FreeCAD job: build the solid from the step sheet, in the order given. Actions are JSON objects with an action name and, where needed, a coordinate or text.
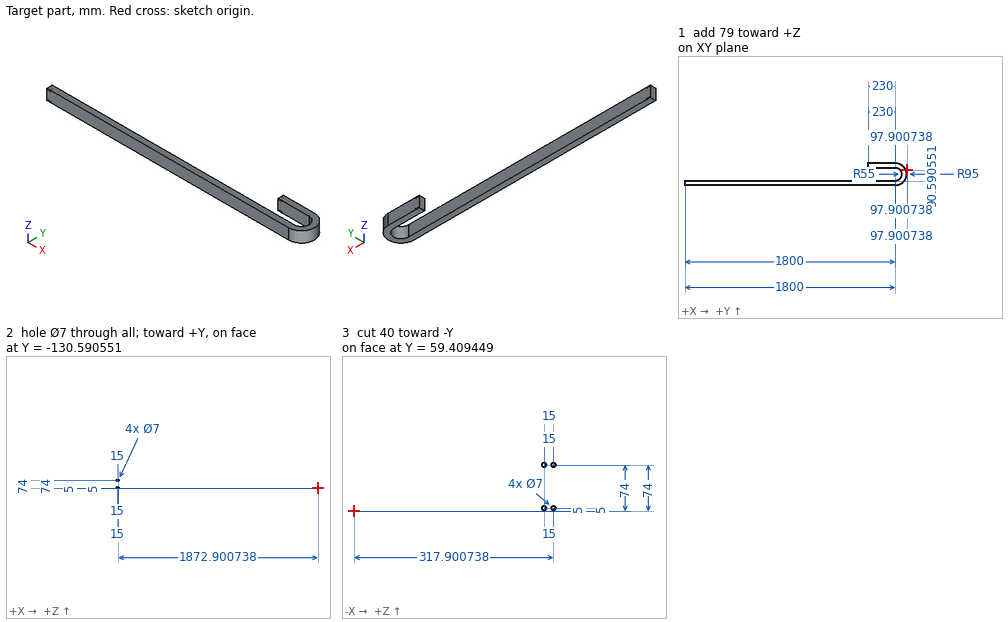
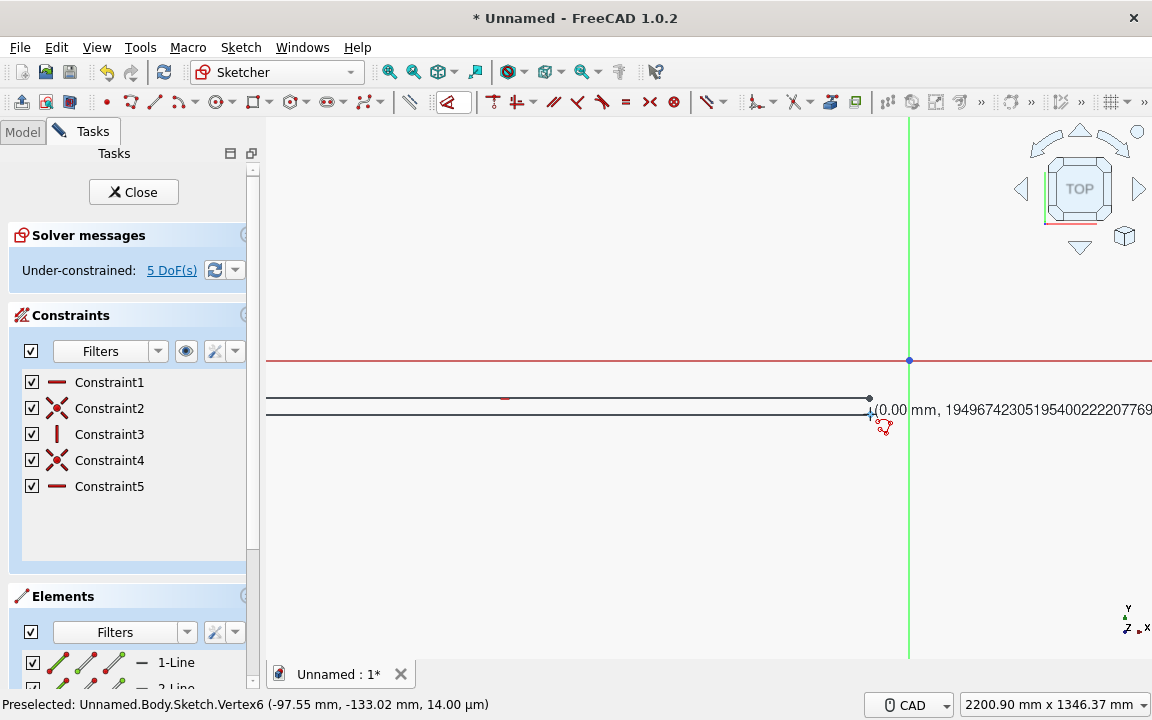
{"action": "left_click", "coordinate": [870, 337]}
{"action": "left_click", "coordinate": [777, 337]}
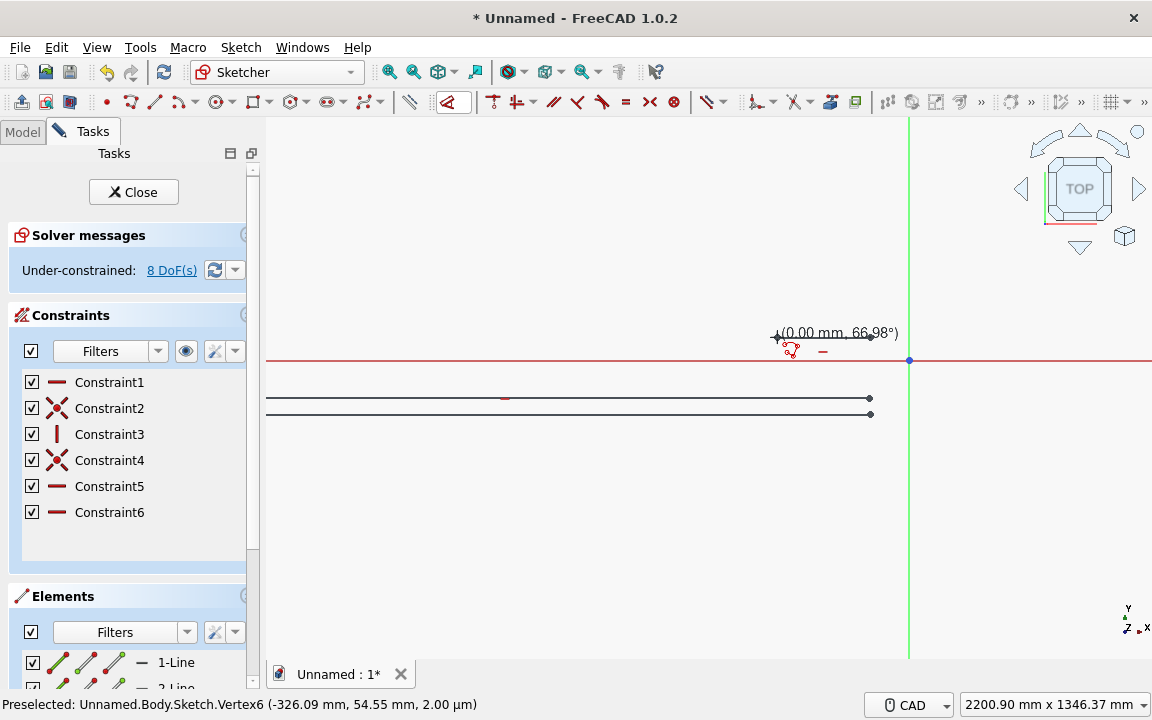
{"action": "scroll", "coordinate": [777, 353], "scroll_direction": "up", "scroll_amount": 4}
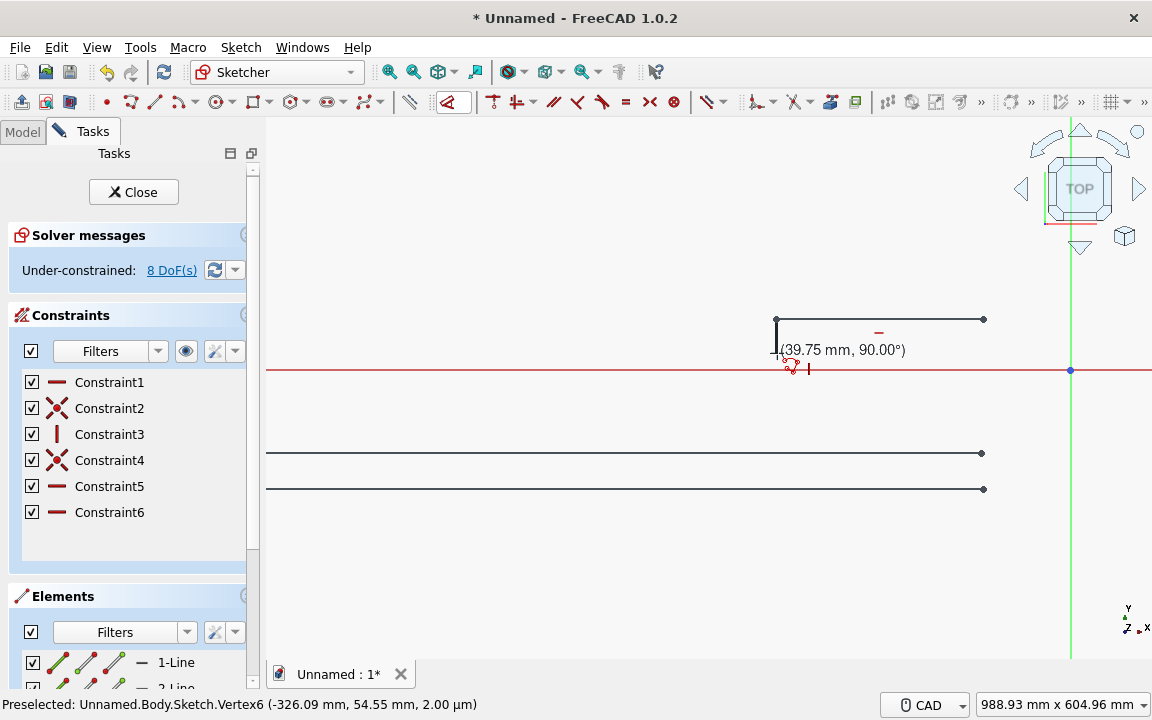
{"action": "left_click", "coordinate": [776, 353]}
{"action": "left_click", "coordinate": [983, 353]}
{"action": "right_click", "coordinate": [983, 353]}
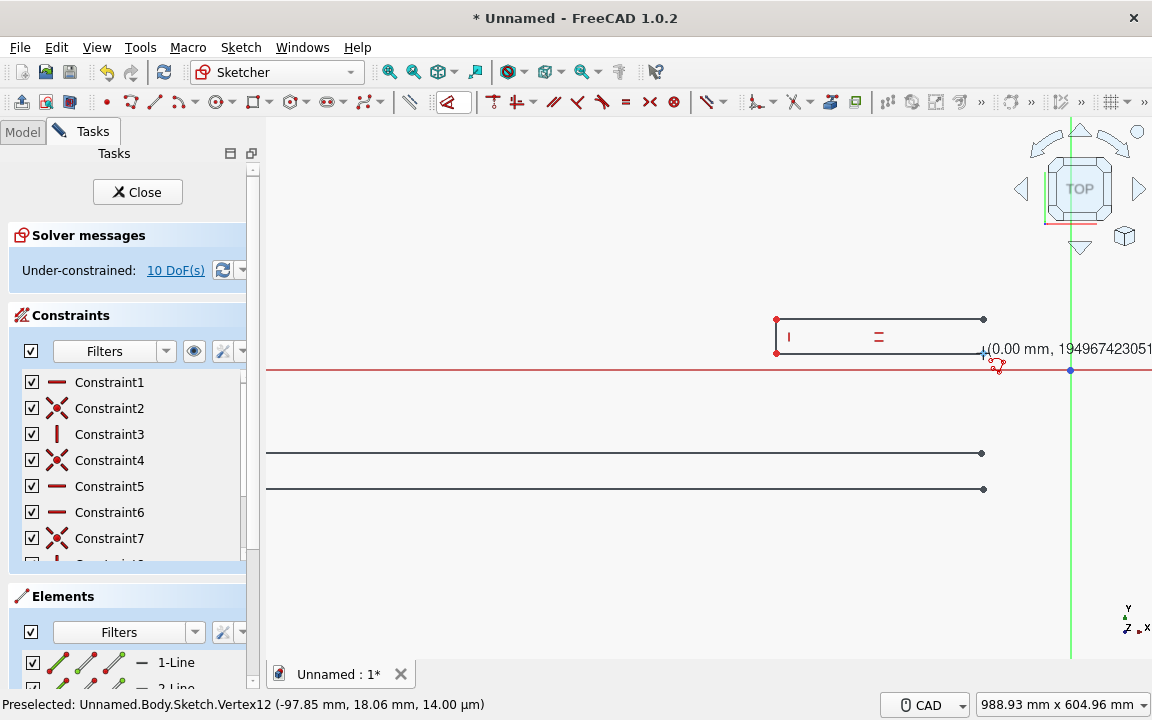
{"action": "key", "text": "g 3 a"}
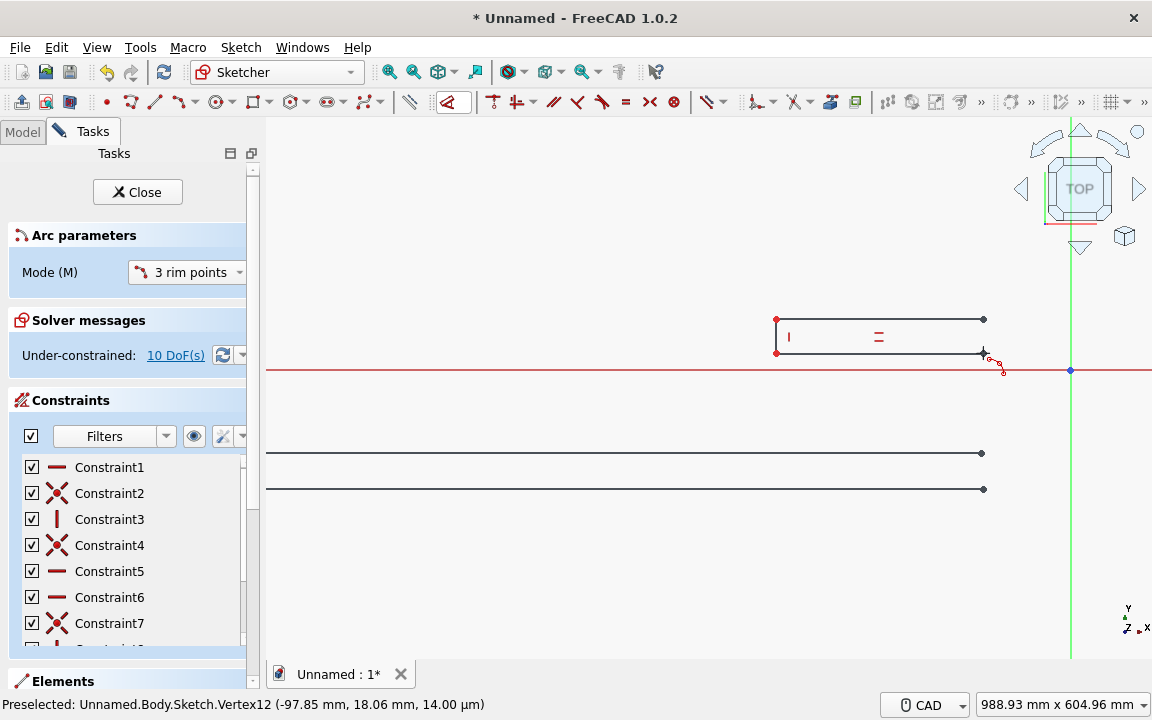
{"action": "left_click", "coordinate": [983, 489]}
{"action": "left_click", "coordinate": [983, 319]}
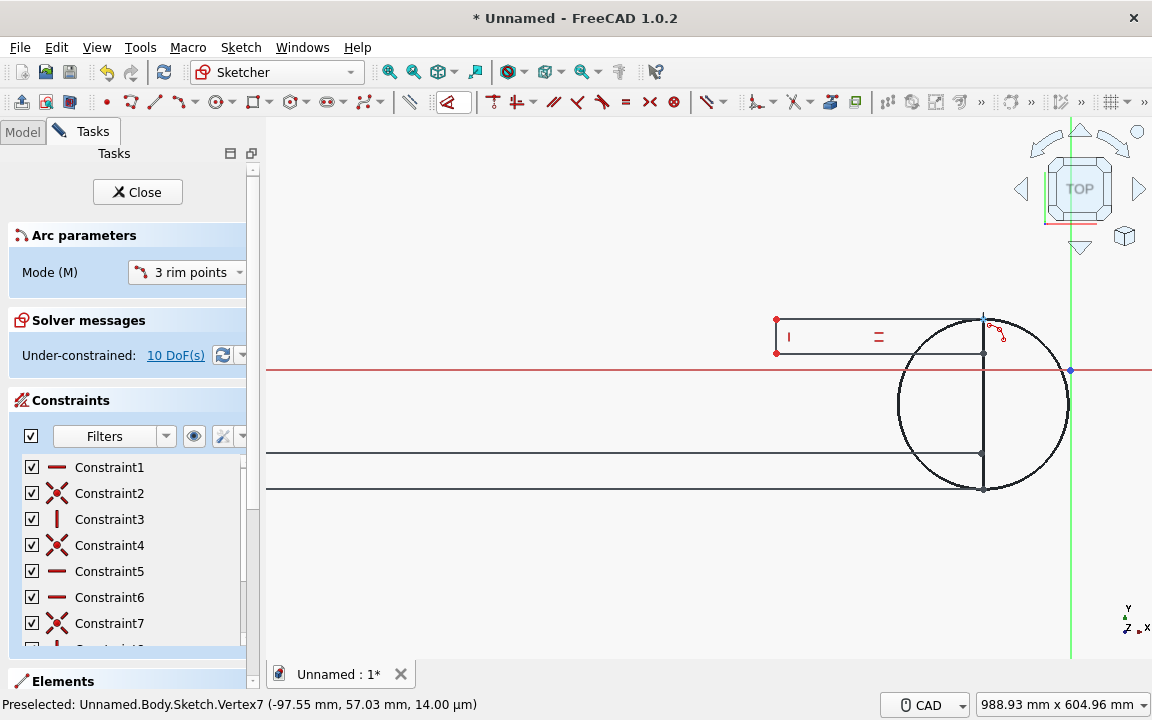
{"action": "scroll", "coordinate": [822, 382], "scroll_direction": "down", "scroll_amount": 6}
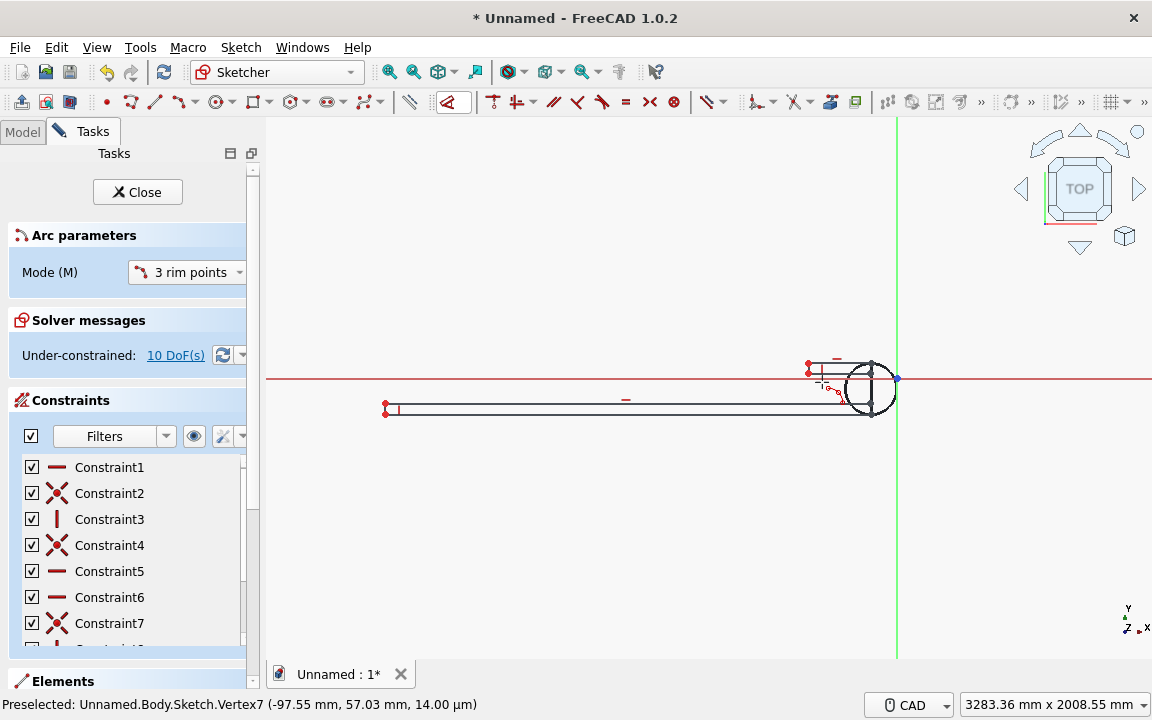
{"action": "scroll", "coordinate": [892, 403], "scroll_direction": "up", "scroll_amount": 6}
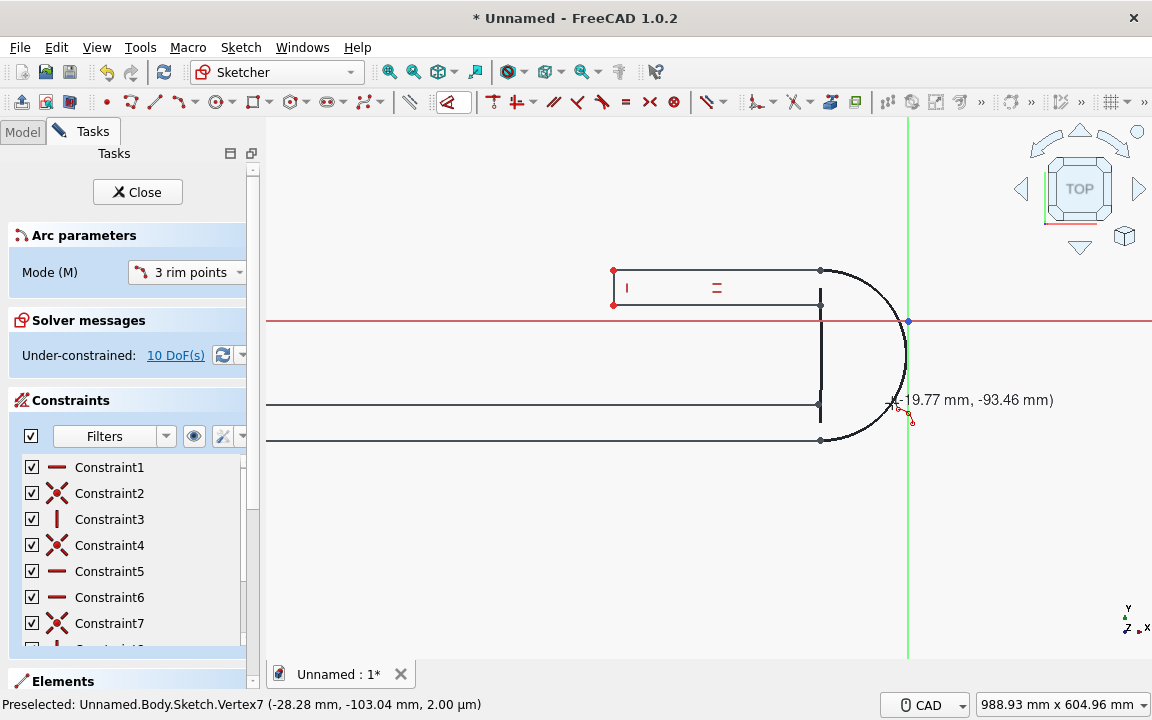
{"action": "left_click", "coordinate": [889, 403]}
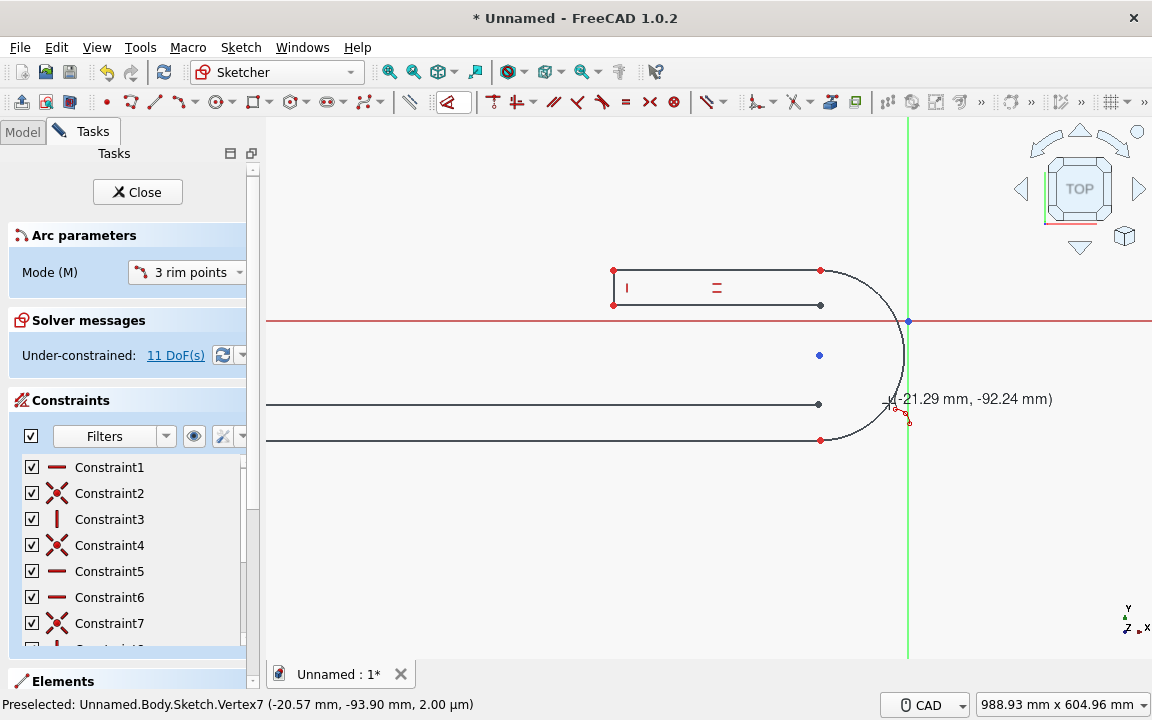
{"action": "left_click", "coordinate": [820, 305]}
{"action": "left_click", "coordinate": [819, 405]}
{"action": "left_click", "coordinate": [867, 368]}
{"action": "key", "text": "Escape"}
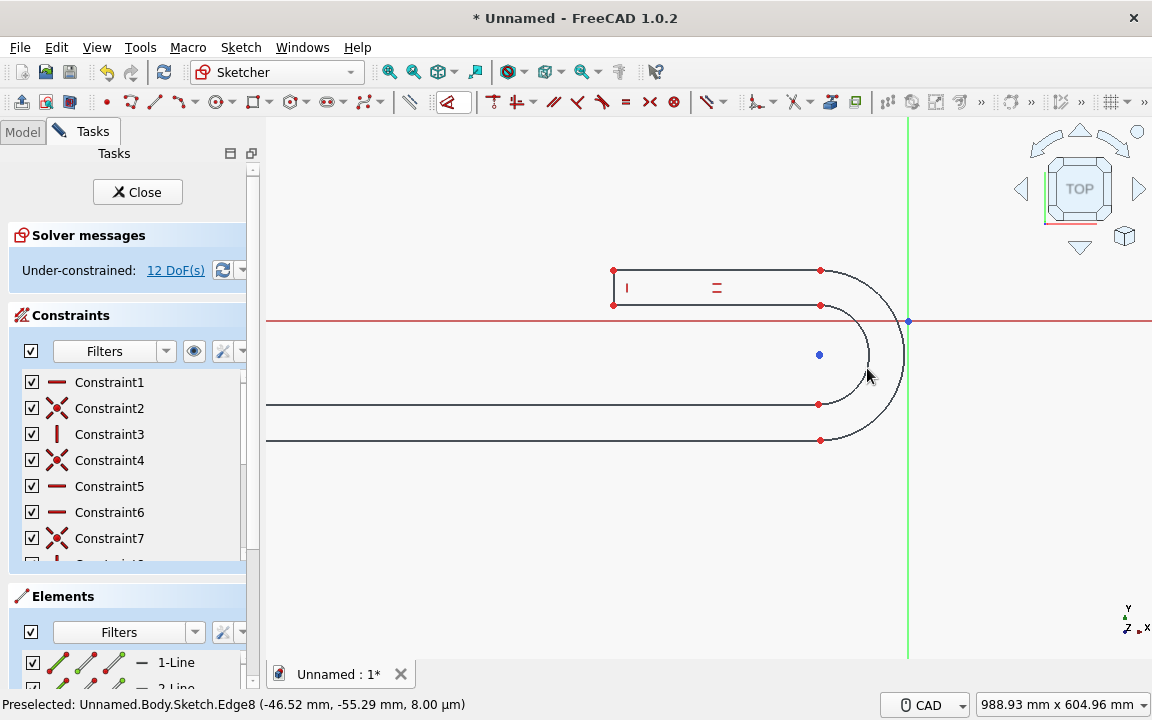
{"action": "left_click", "coordinate": [888, 405]}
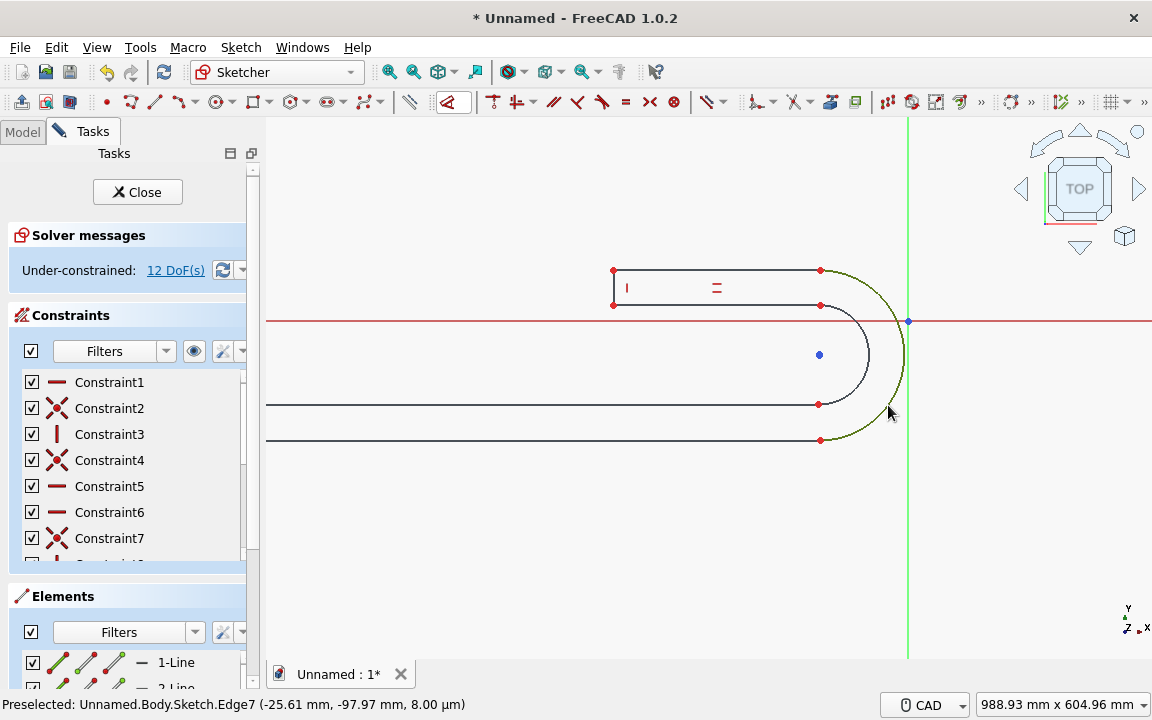
{"action": "left_click", "coordinate": [859, 385]}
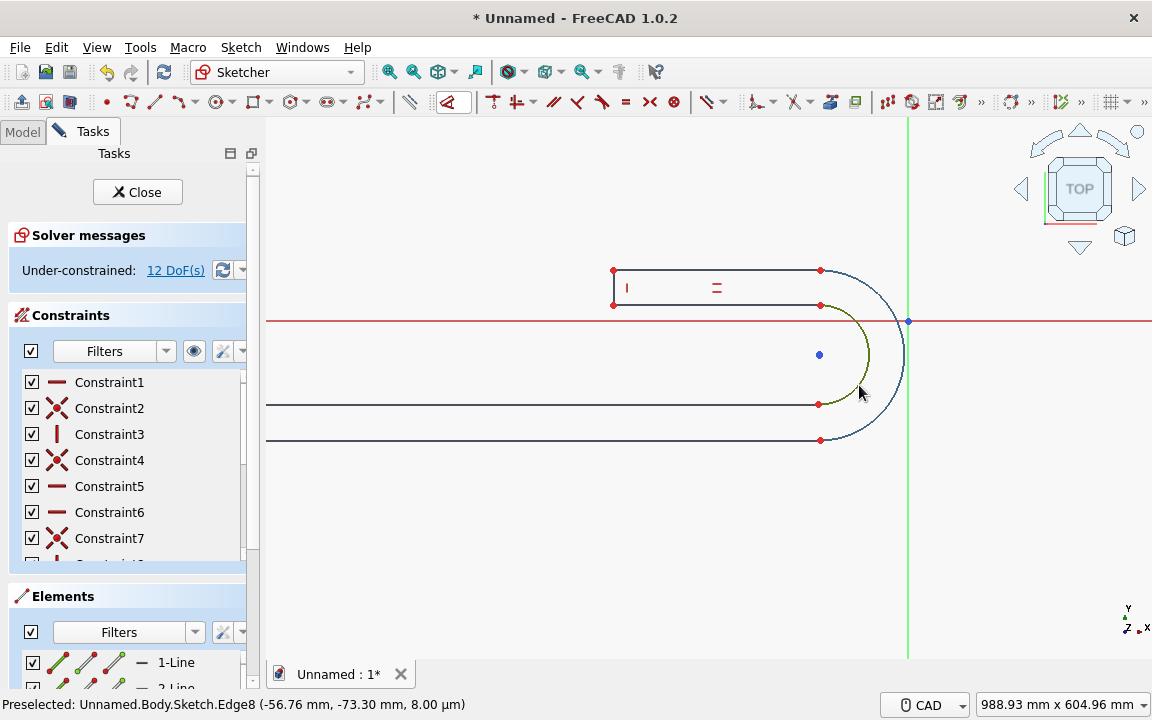
{"action": "left_click", "coordinate": [494, 102]}